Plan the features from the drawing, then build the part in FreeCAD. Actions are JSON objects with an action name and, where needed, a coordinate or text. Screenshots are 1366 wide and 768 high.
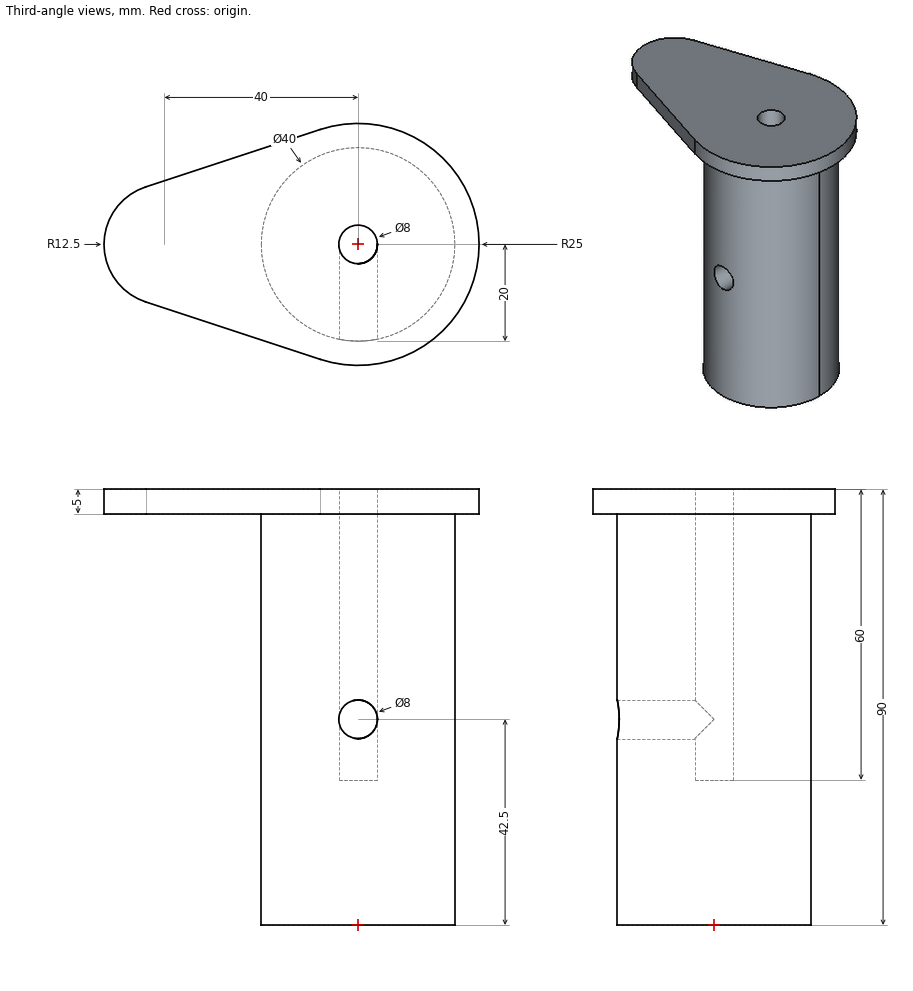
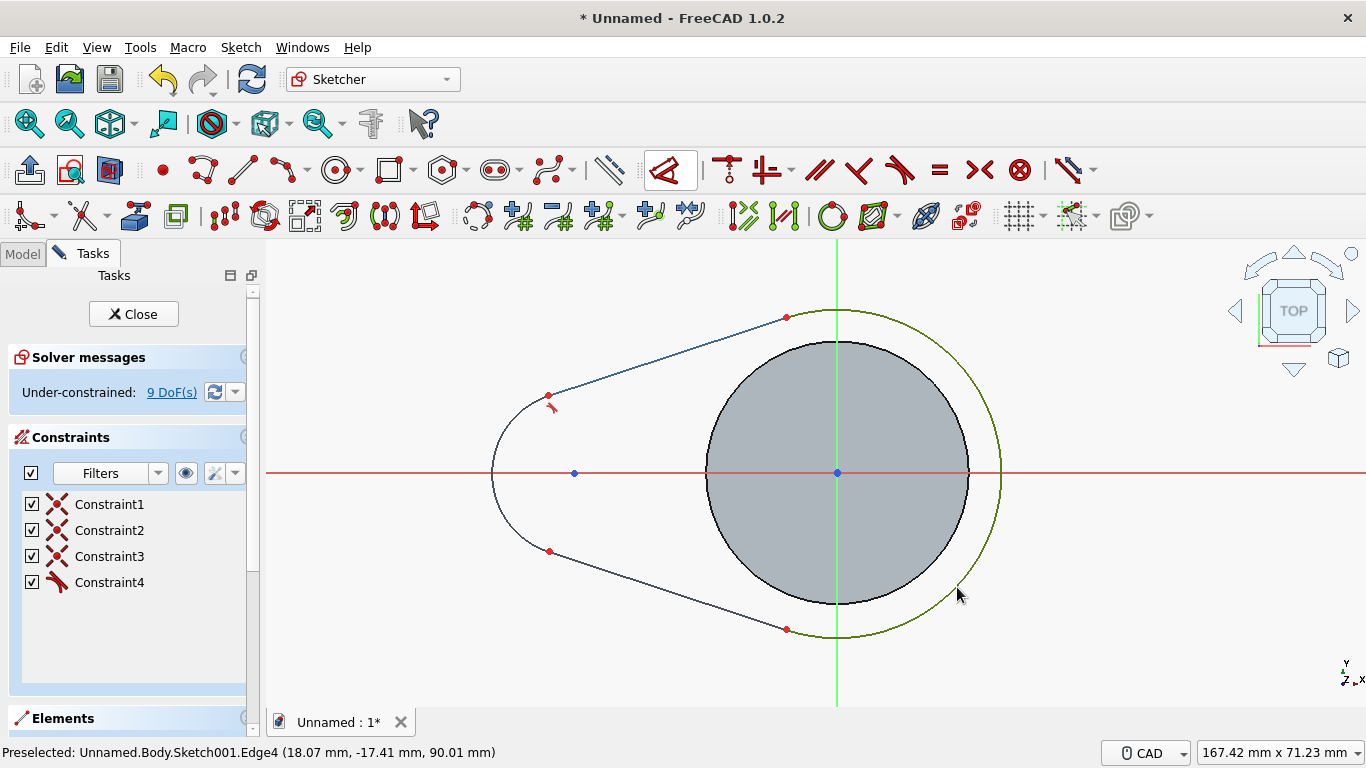
{"action": "left_click", "coordinate": [900, 170]}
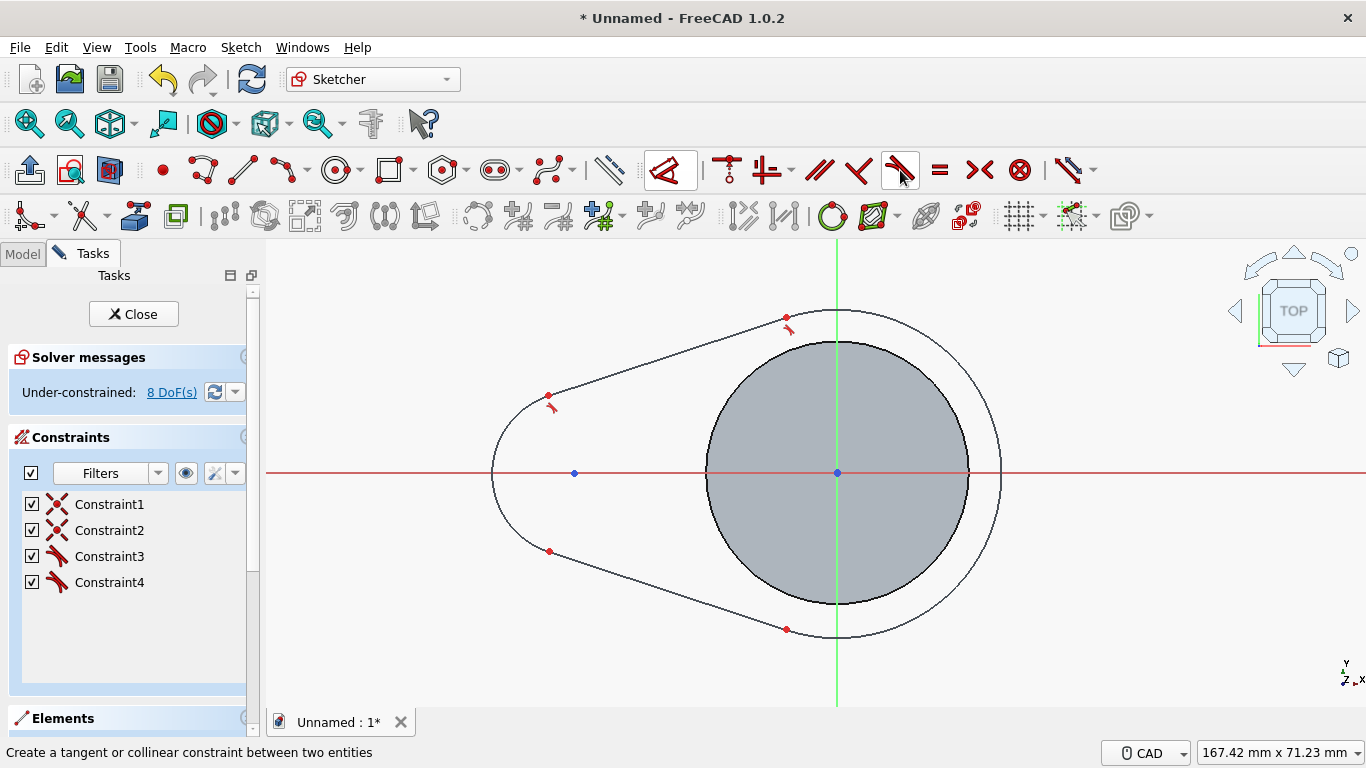
{"action": "left_click", "coordinate": [620, 575]}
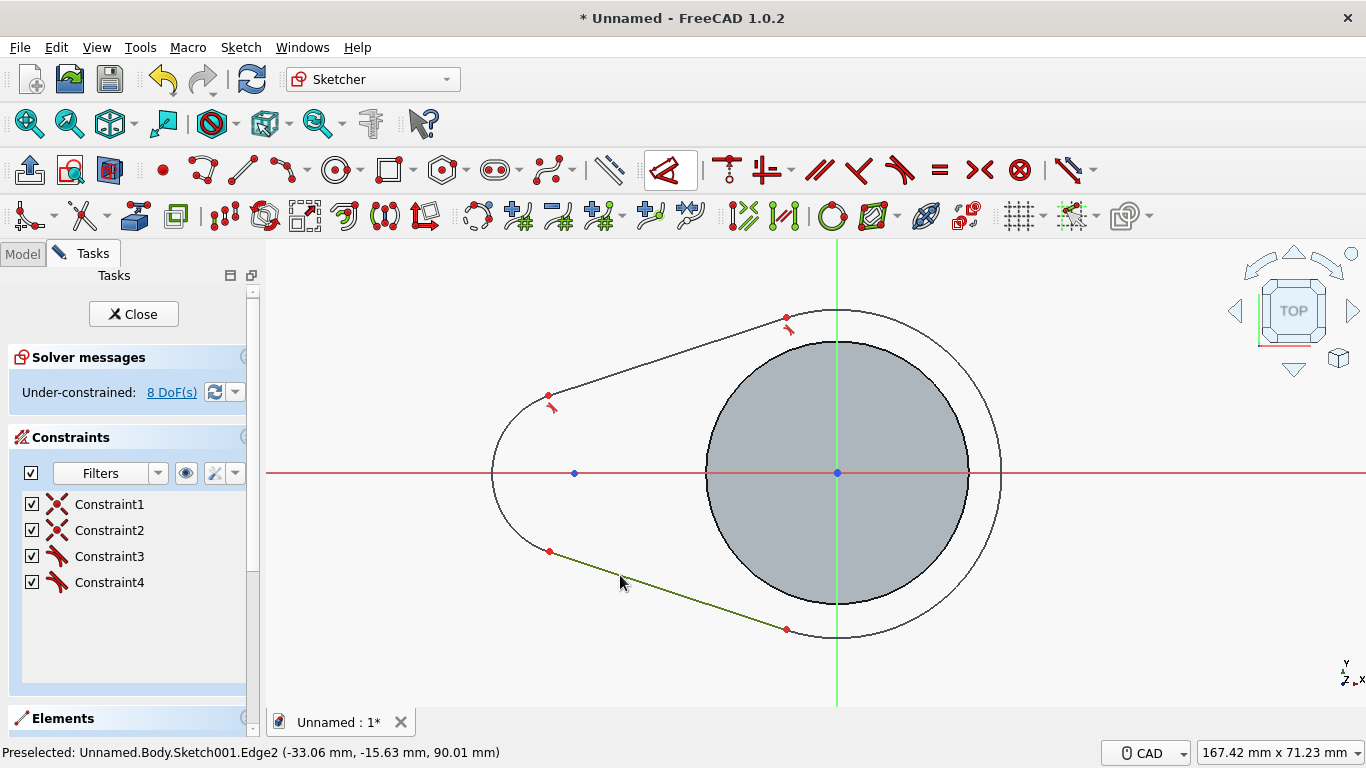
{"action": "left_click", "coordinate": [502, 435]}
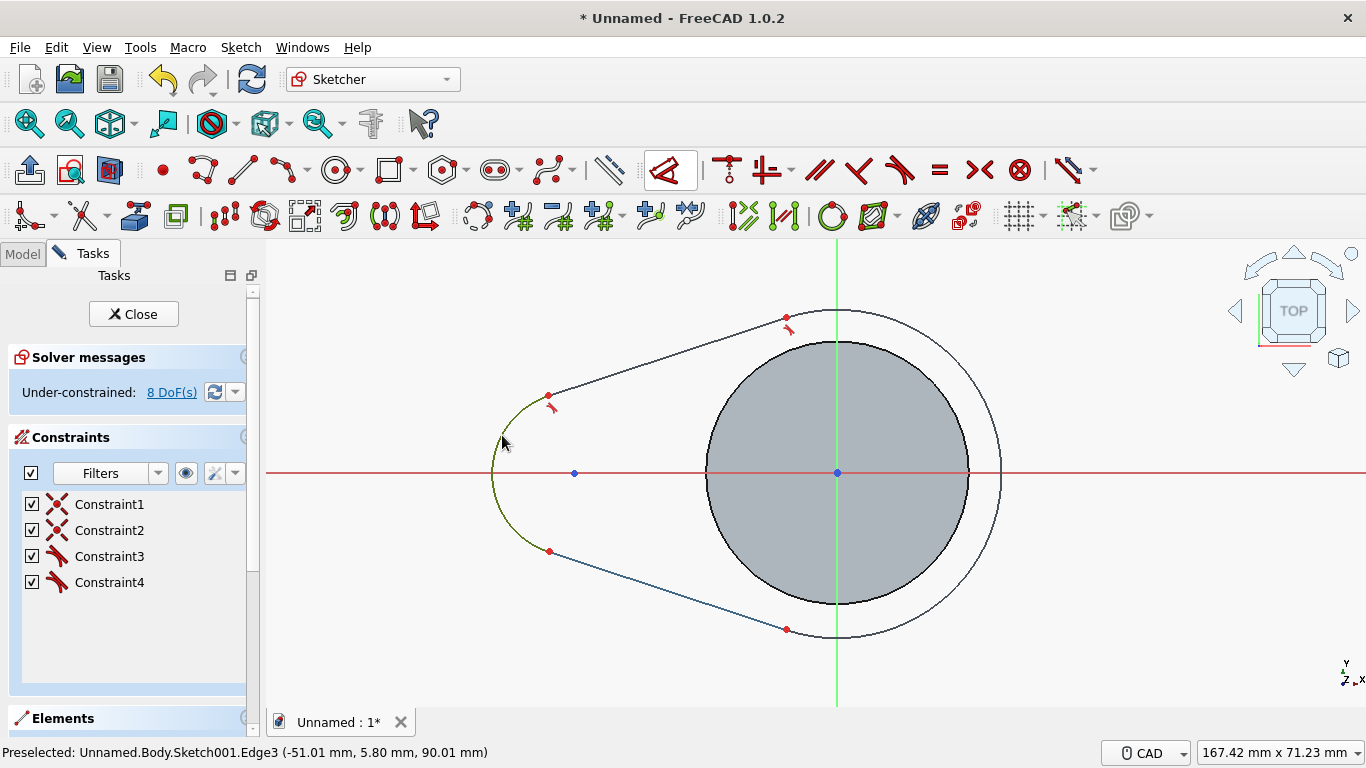
{"action": "key", "text": "t"}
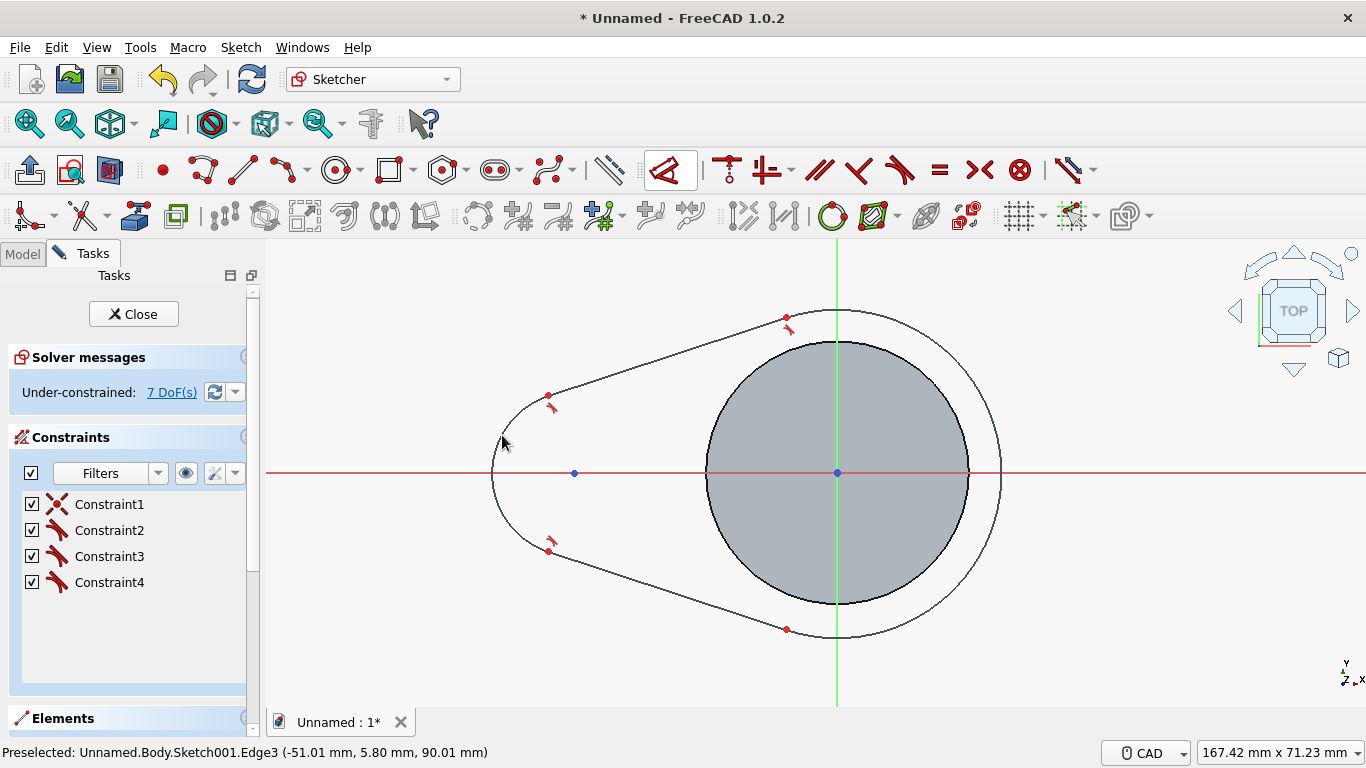
{"action": "left_click", "coordinate": [620, 575]}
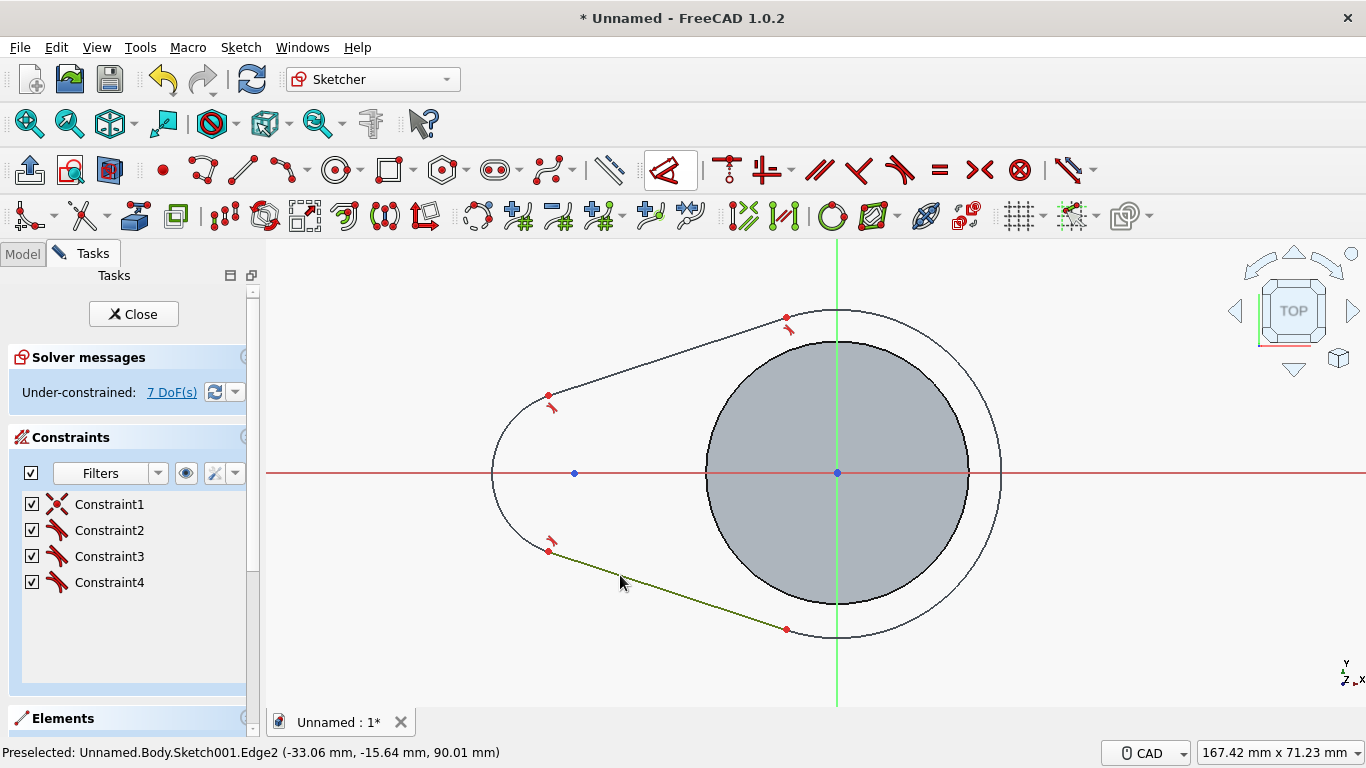
{"action": "left_click", "coordinate": [957, 587]}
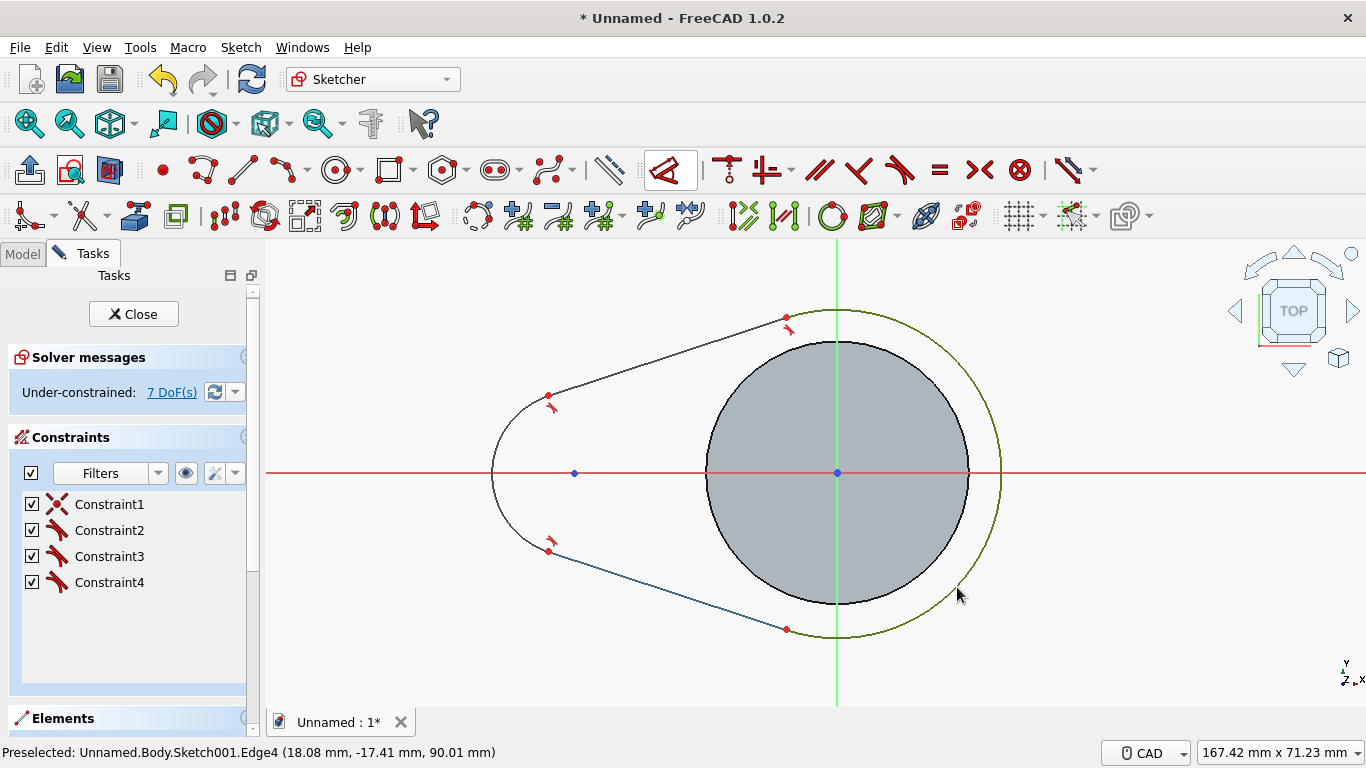
{"action": "left_click", "coordinate": [900, 170]}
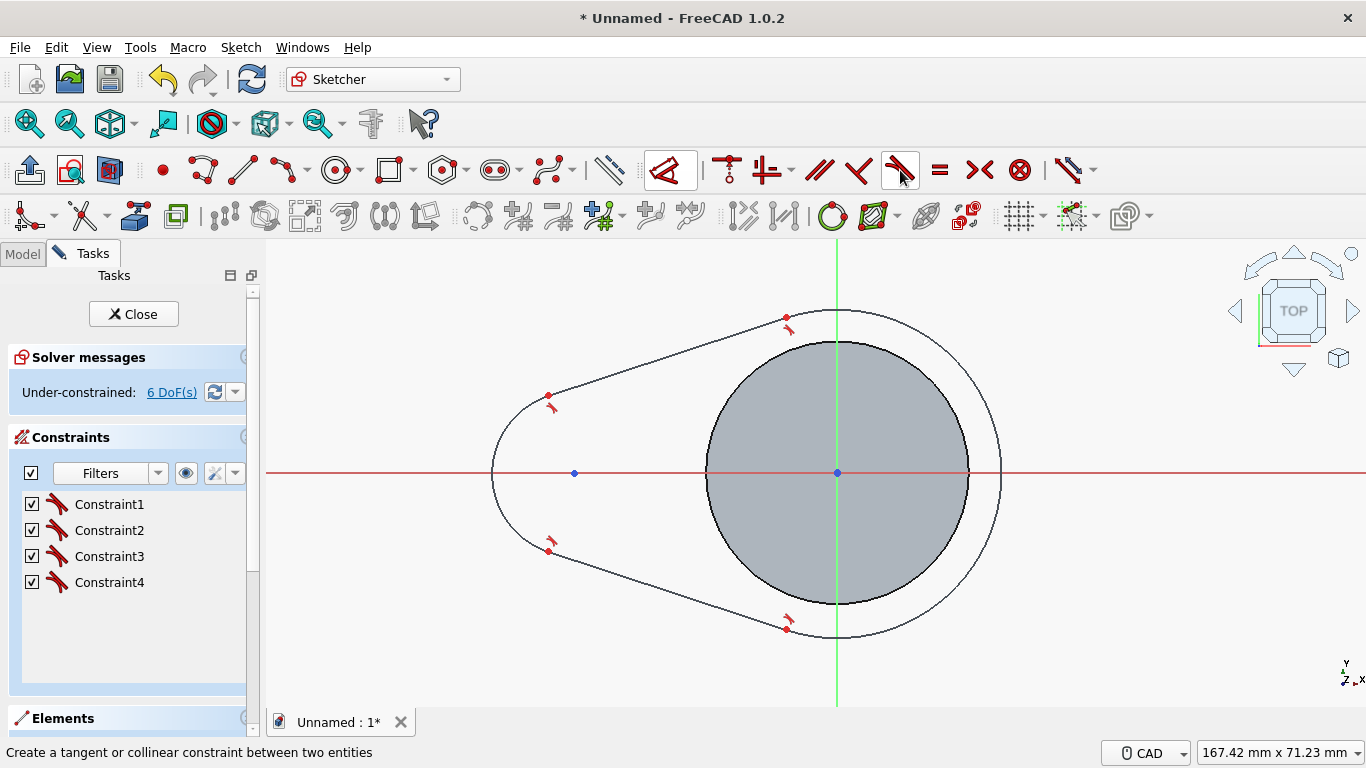
{"action": "left_click_drag", "start_coordinate": [827, 463], "coordinate": [847, 484]}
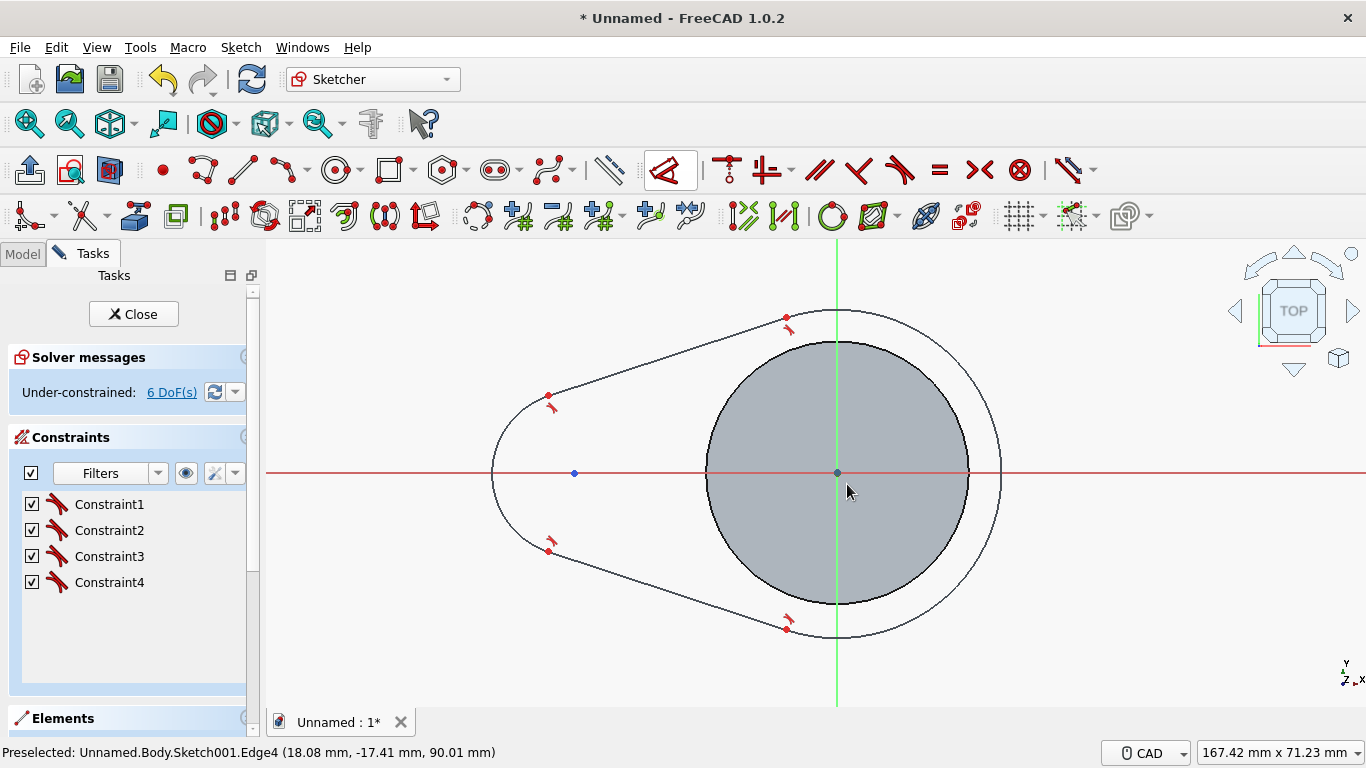
{"action": "left_click", "coordinate": [728, 170]}